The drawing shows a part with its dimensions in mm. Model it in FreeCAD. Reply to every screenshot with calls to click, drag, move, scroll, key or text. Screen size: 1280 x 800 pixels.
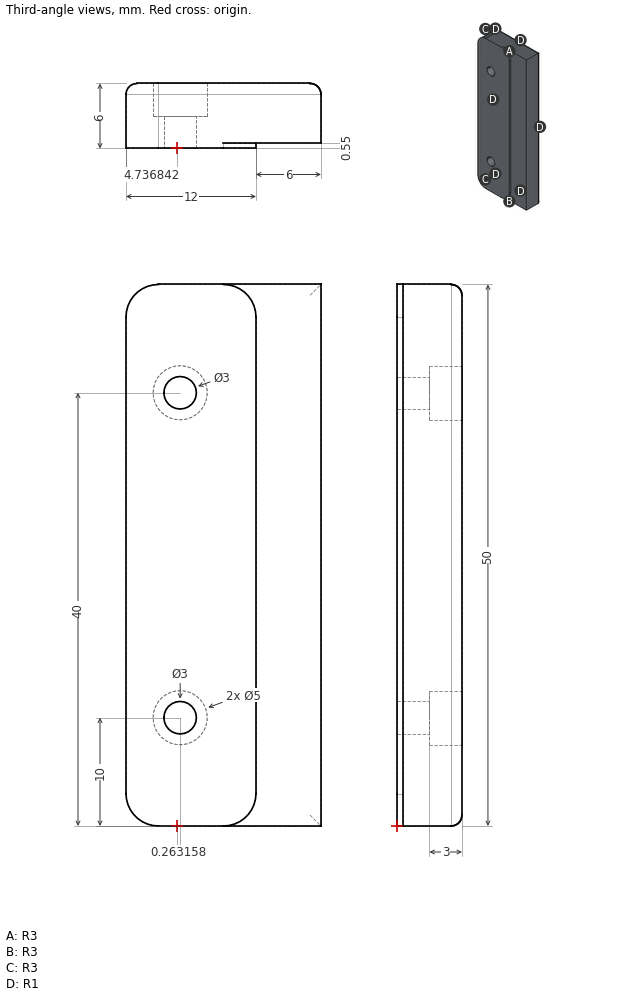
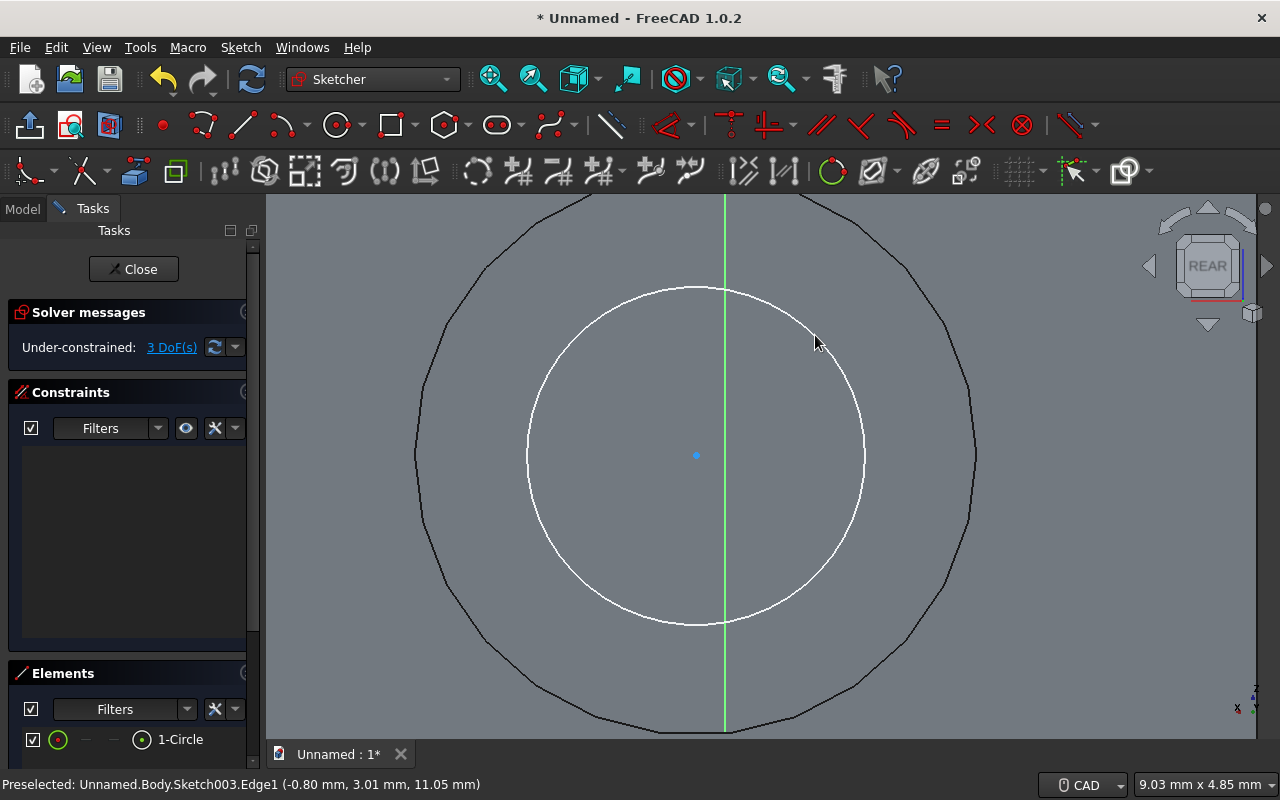
click(666, 126)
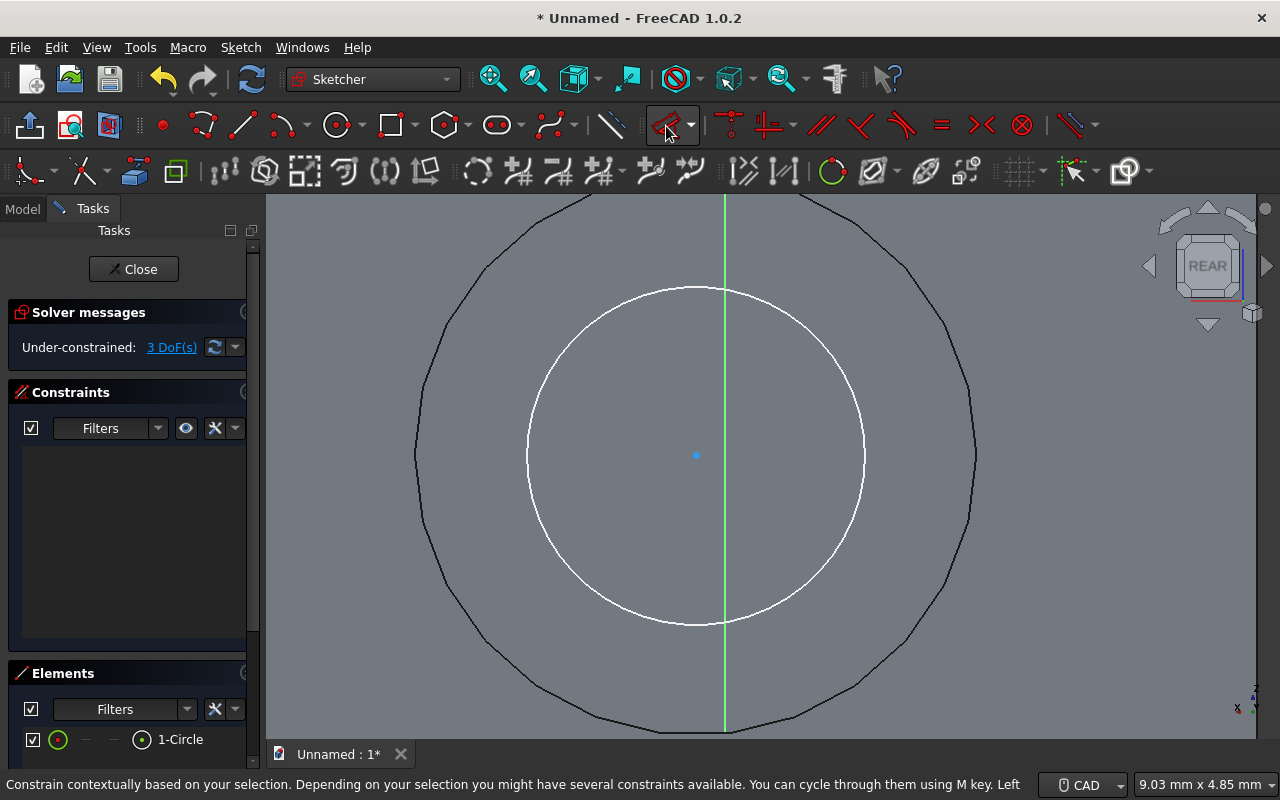
click(815, 336)
click(838, 313)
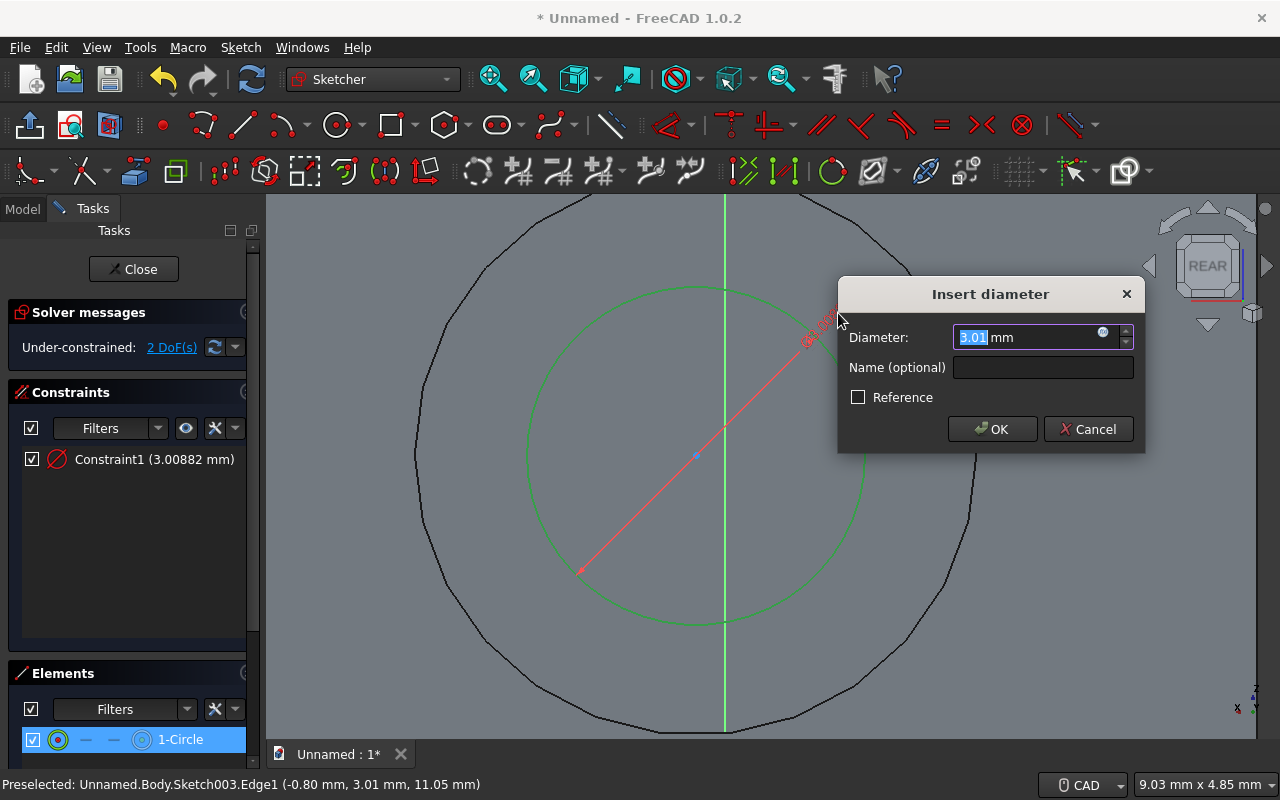
text(3)
key(Return)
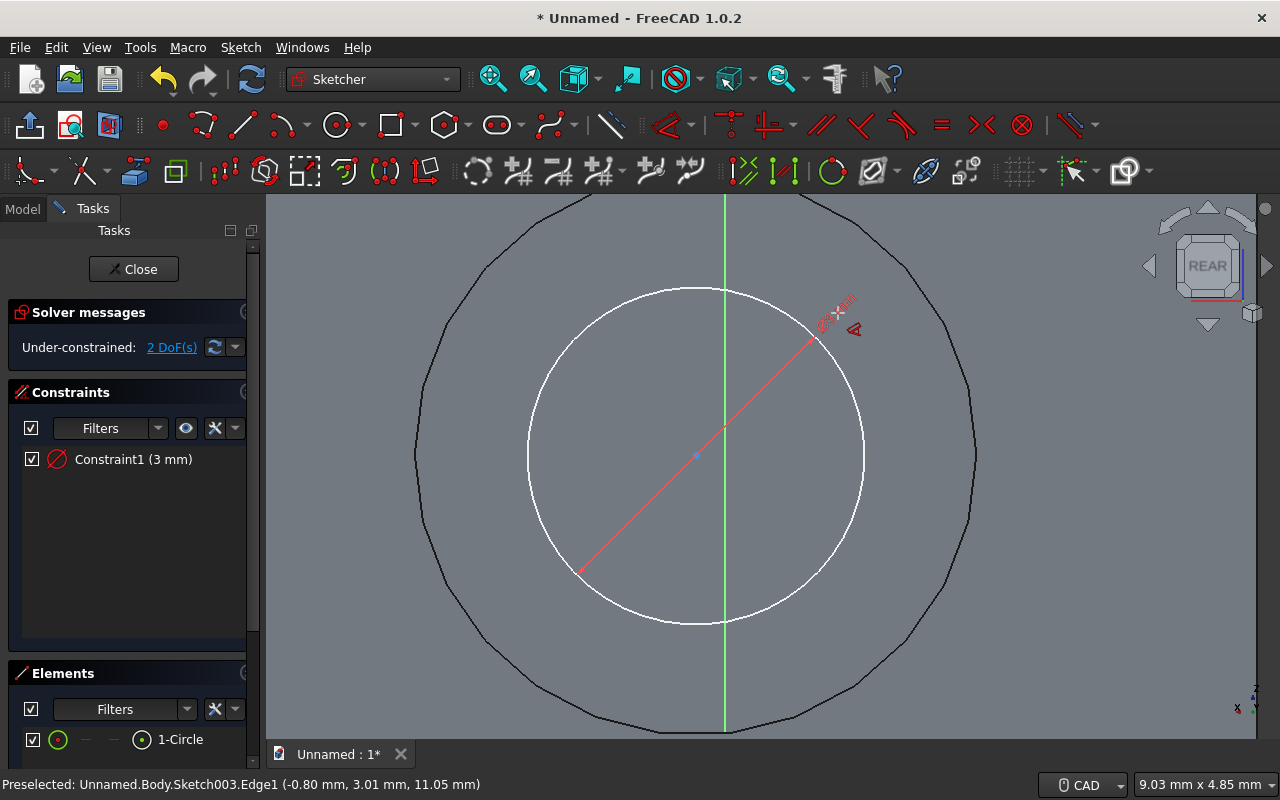
click(696, 456)
click(759, 584)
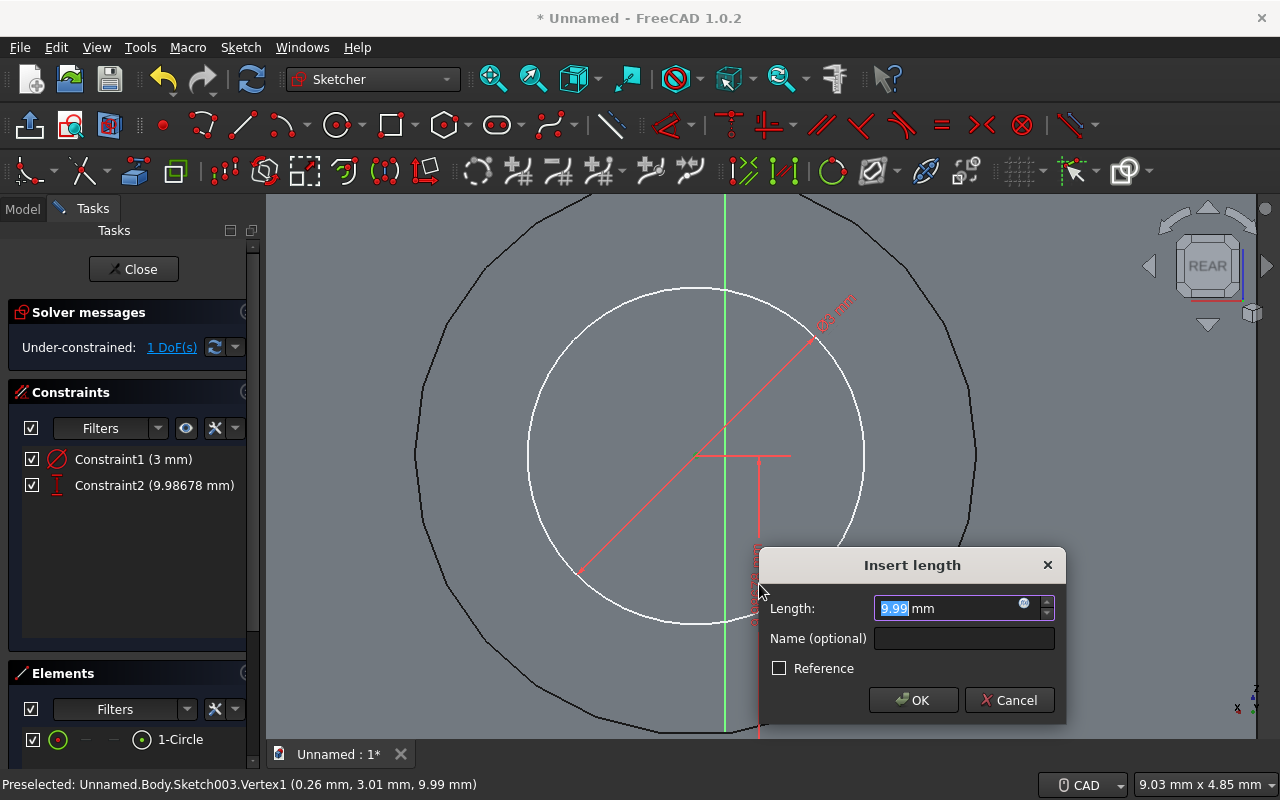
text(10)
key(Return)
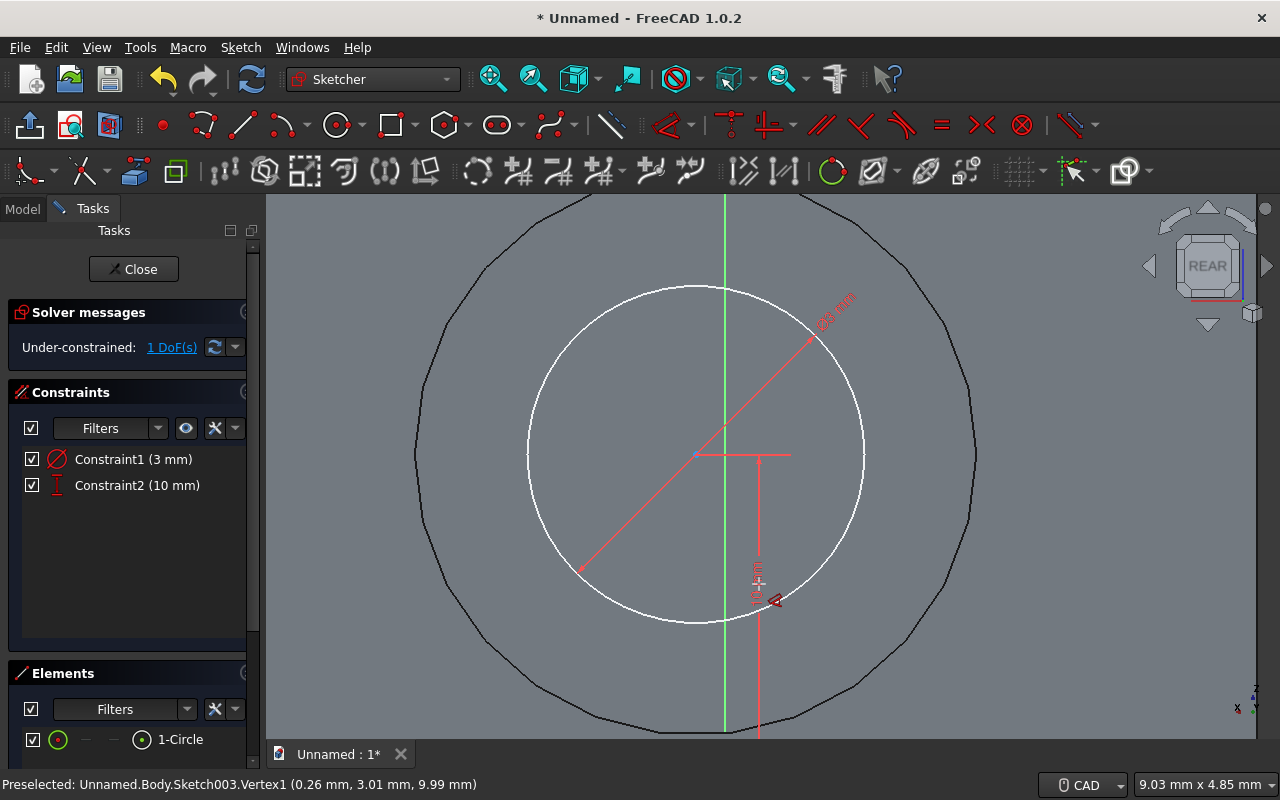
scroll(696, 455, up, 2)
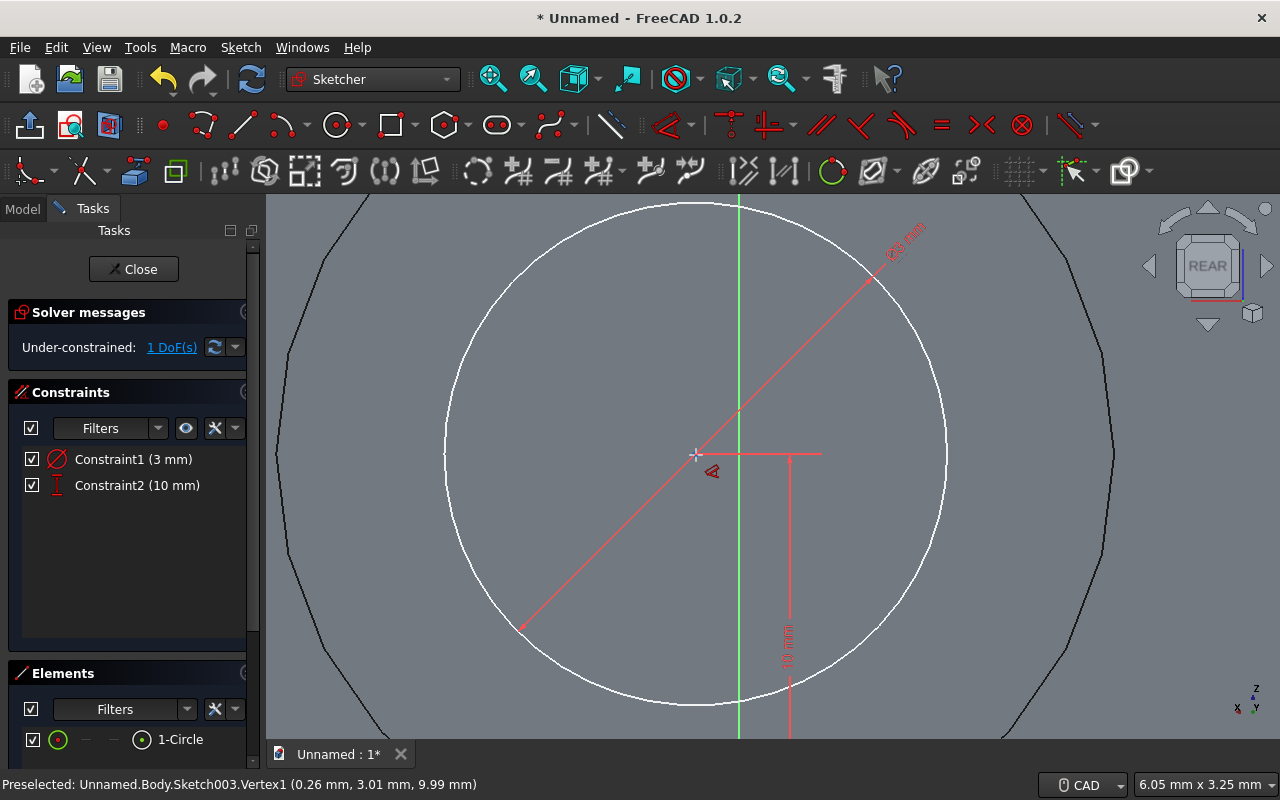
click(696, 454)
click(718, 420)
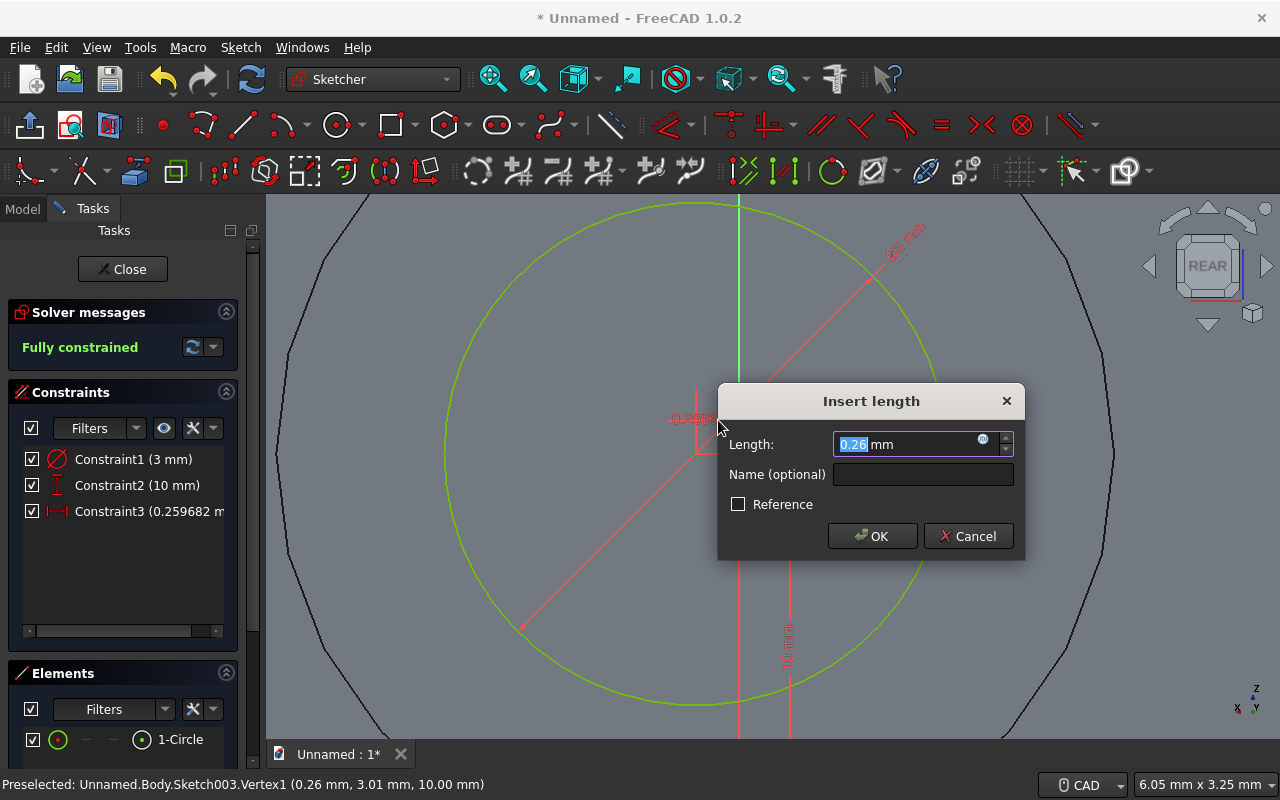
text(0.263158)
key(Return)
key(Escape)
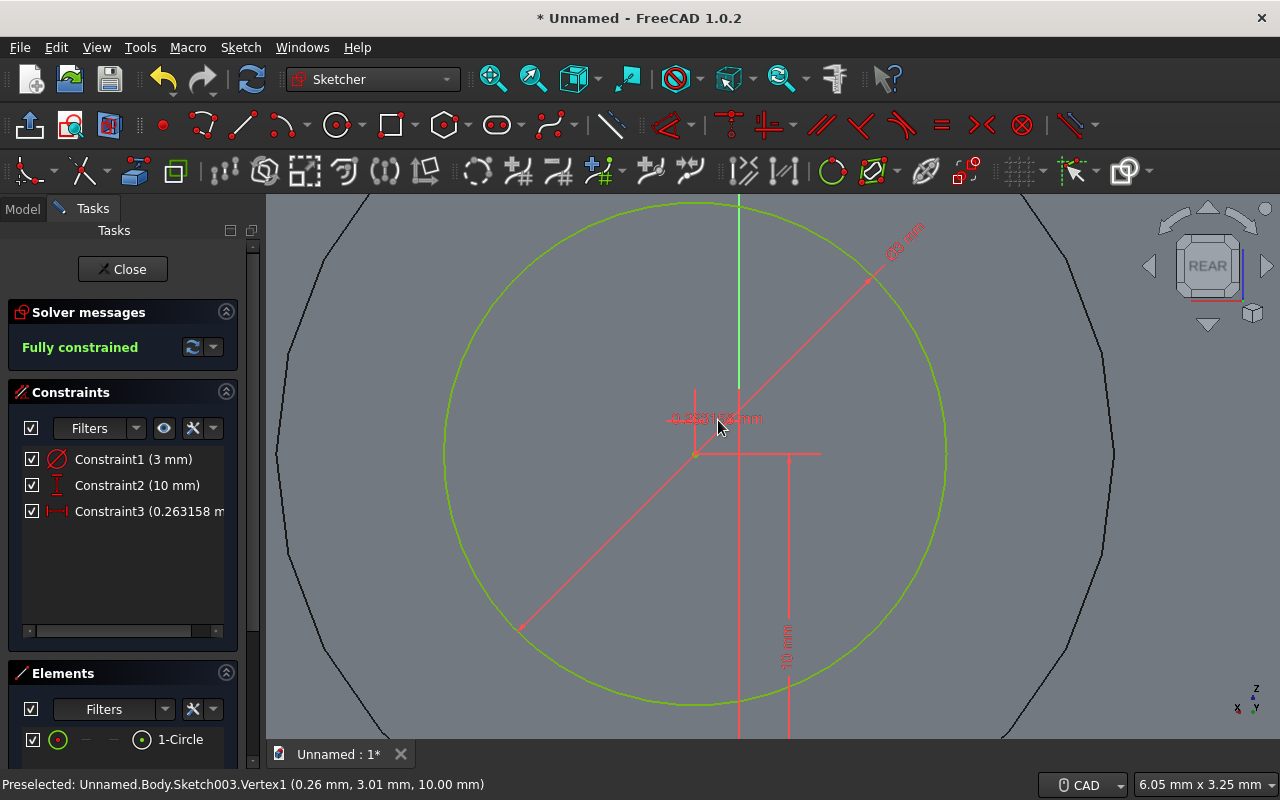
click(123, 269)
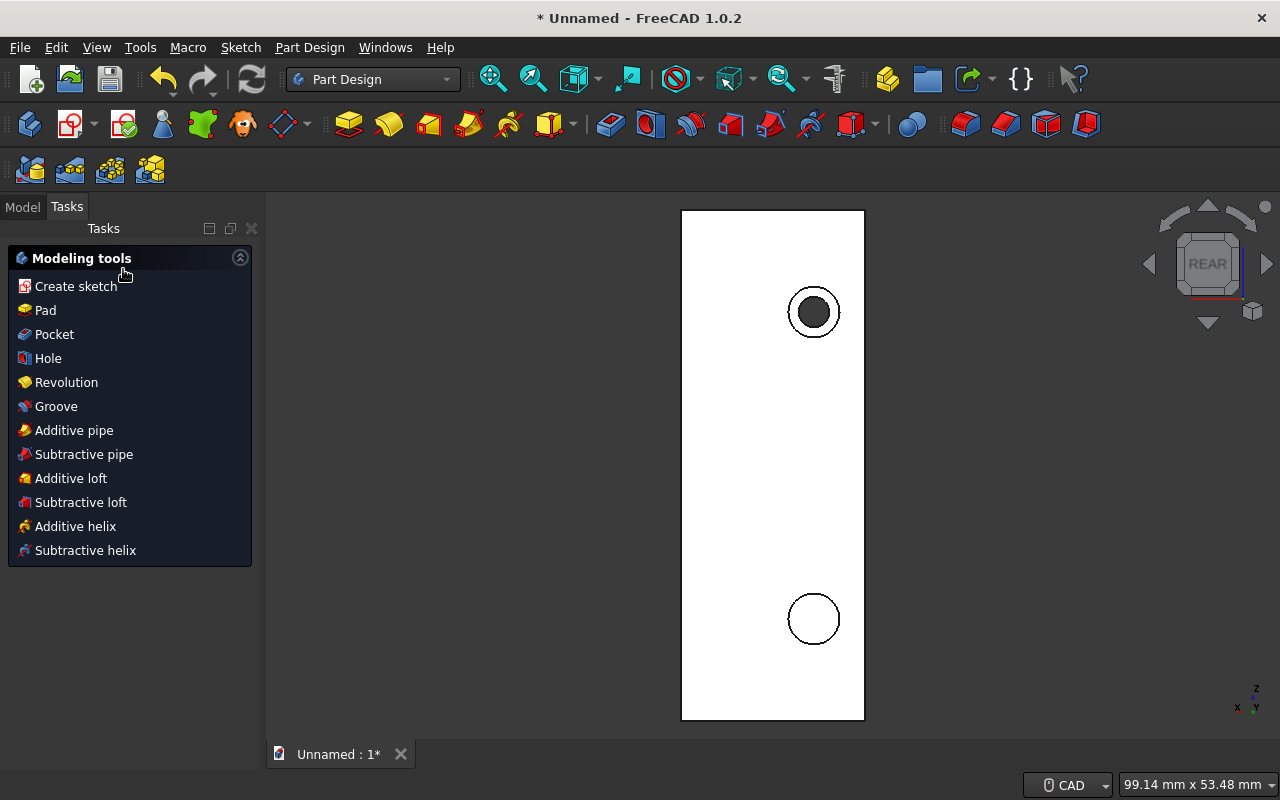
click(612, 124)